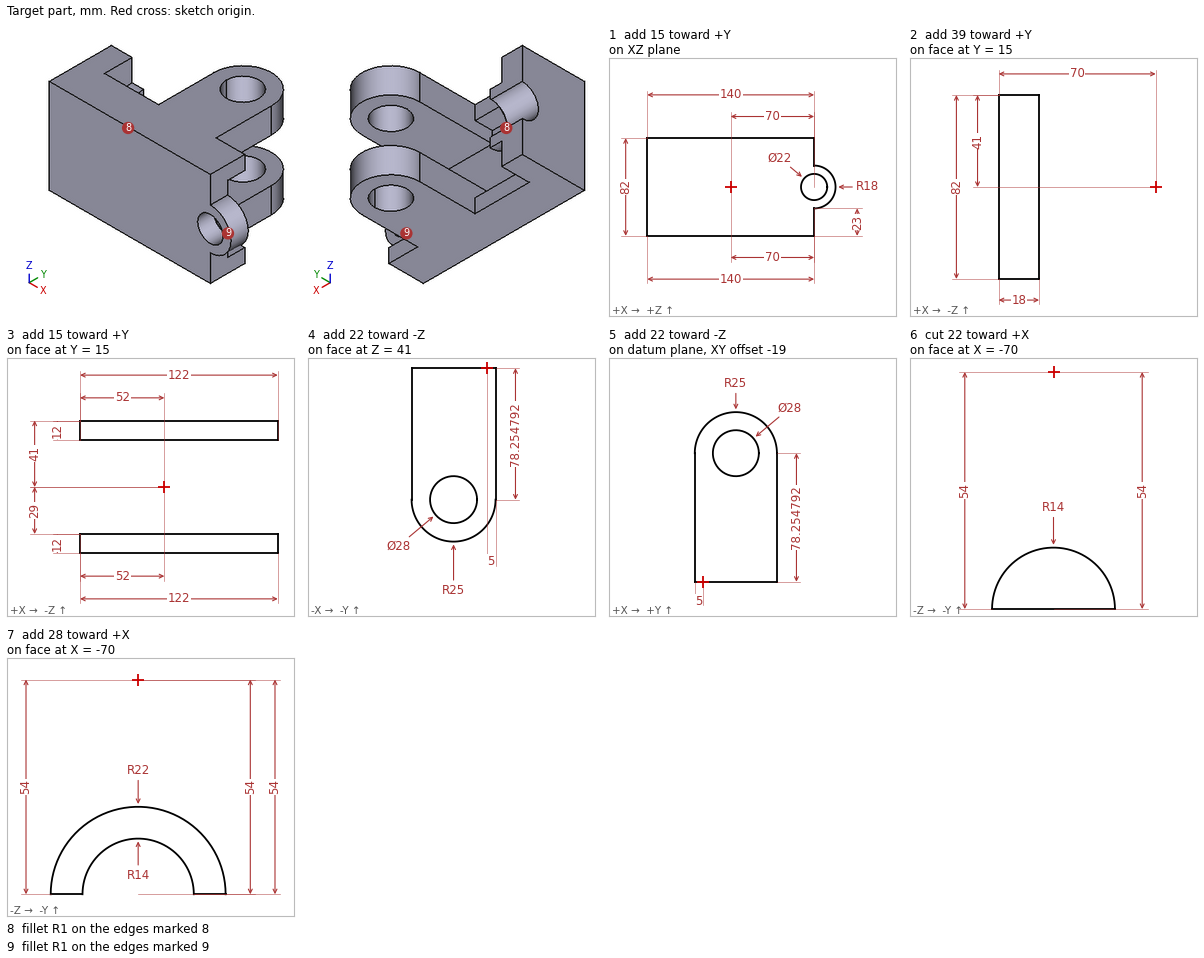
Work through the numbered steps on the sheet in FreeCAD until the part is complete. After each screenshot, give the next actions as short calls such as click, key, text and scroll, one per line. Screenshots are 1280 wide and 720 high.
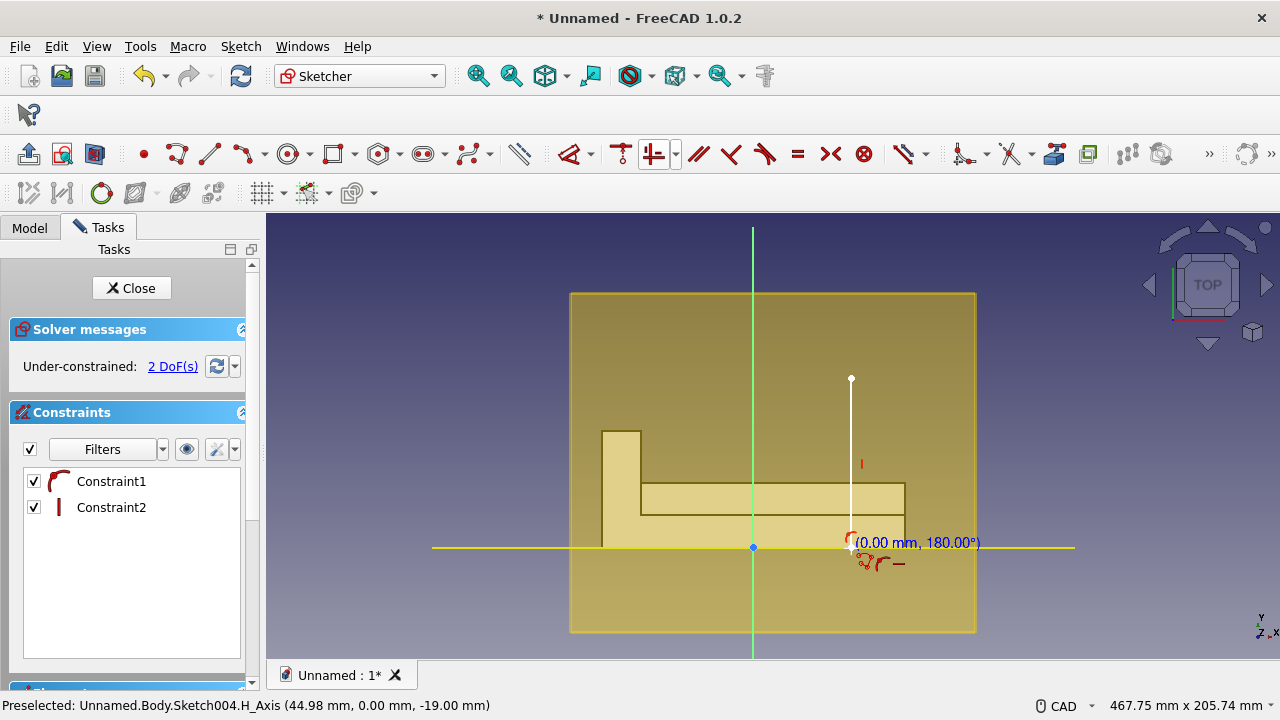
scroll(743, 548, up, 2)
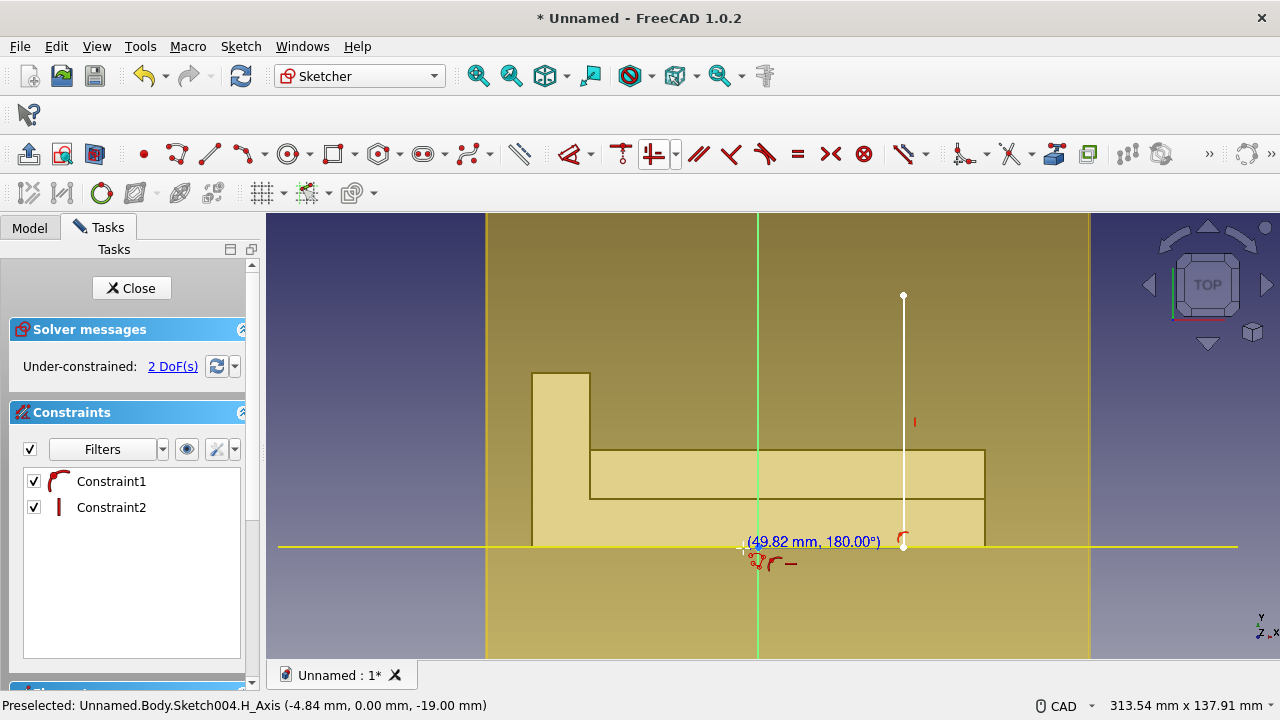
click(742, 538)
click(742, 294)
right_click(742, 294)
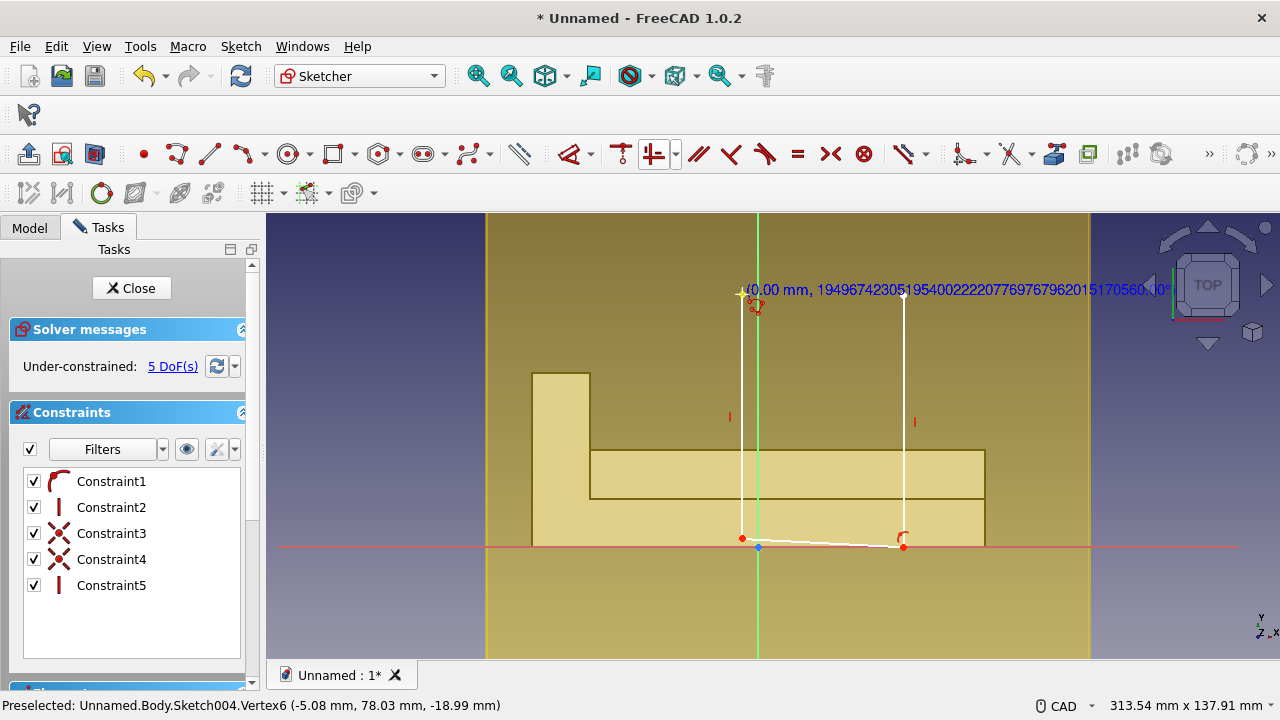
click(242, 154)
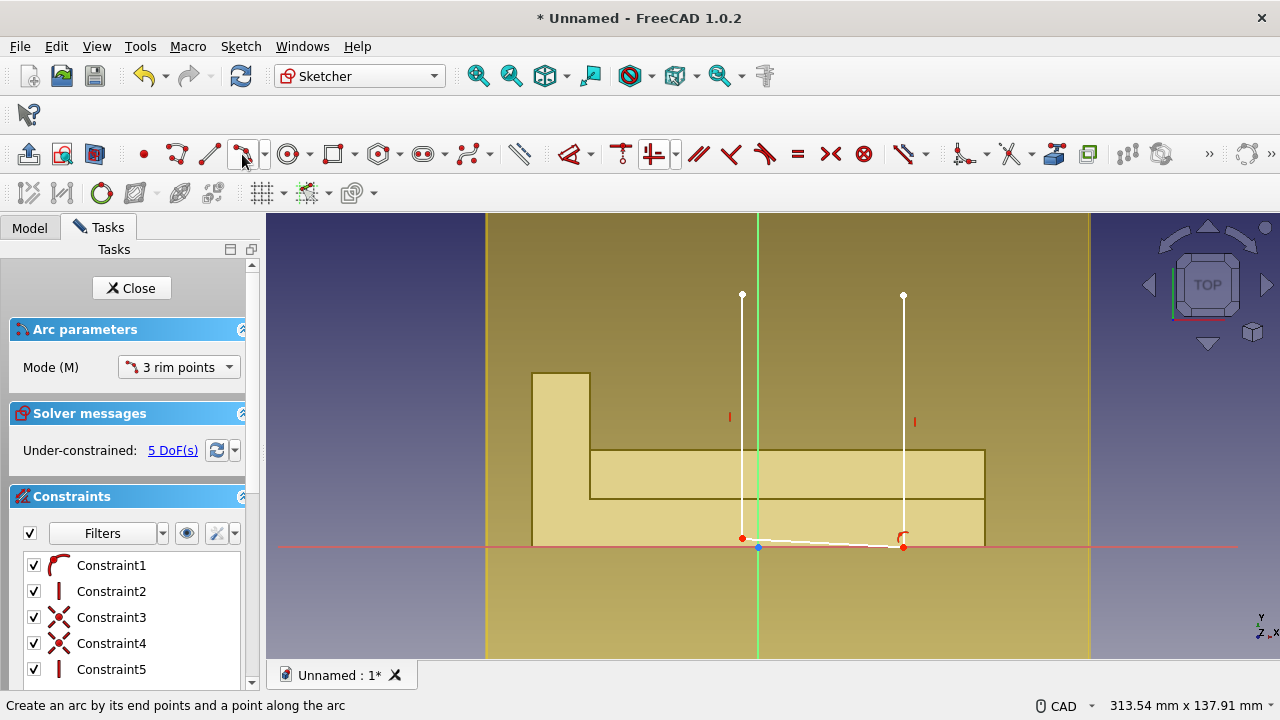
click(742, 295)
click(904, 296)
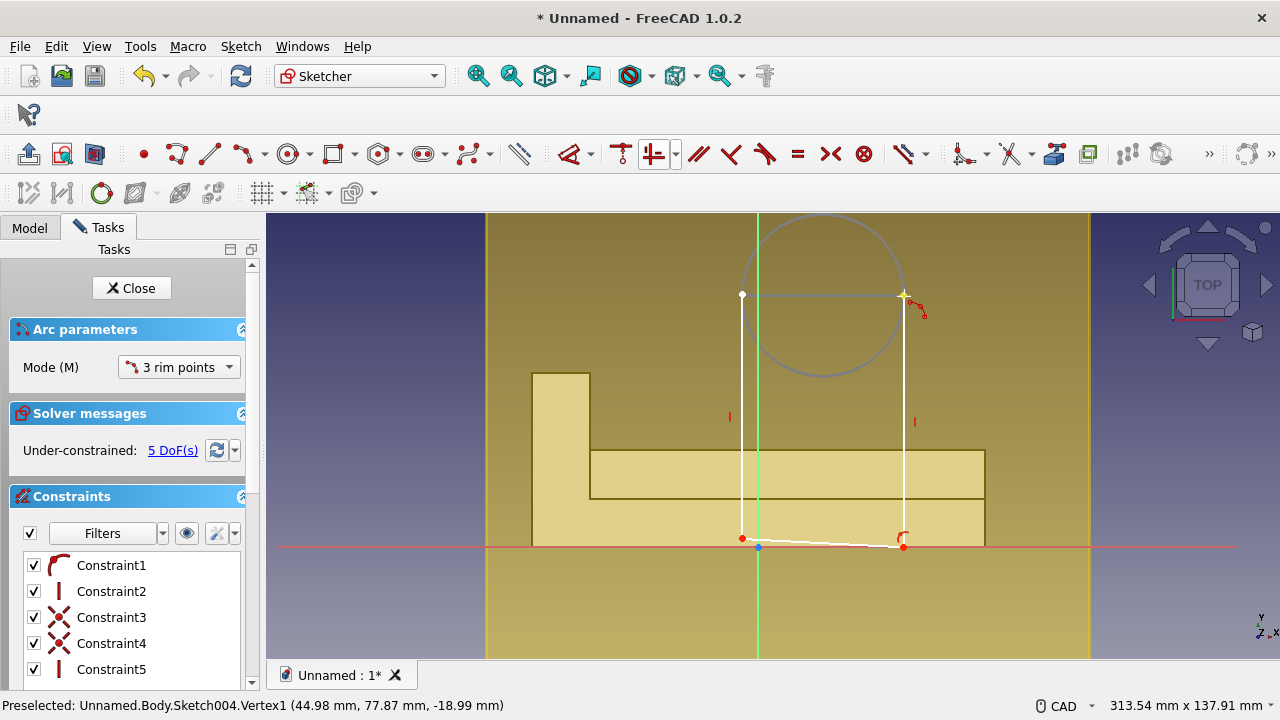
scroll(294, 631, down, 1)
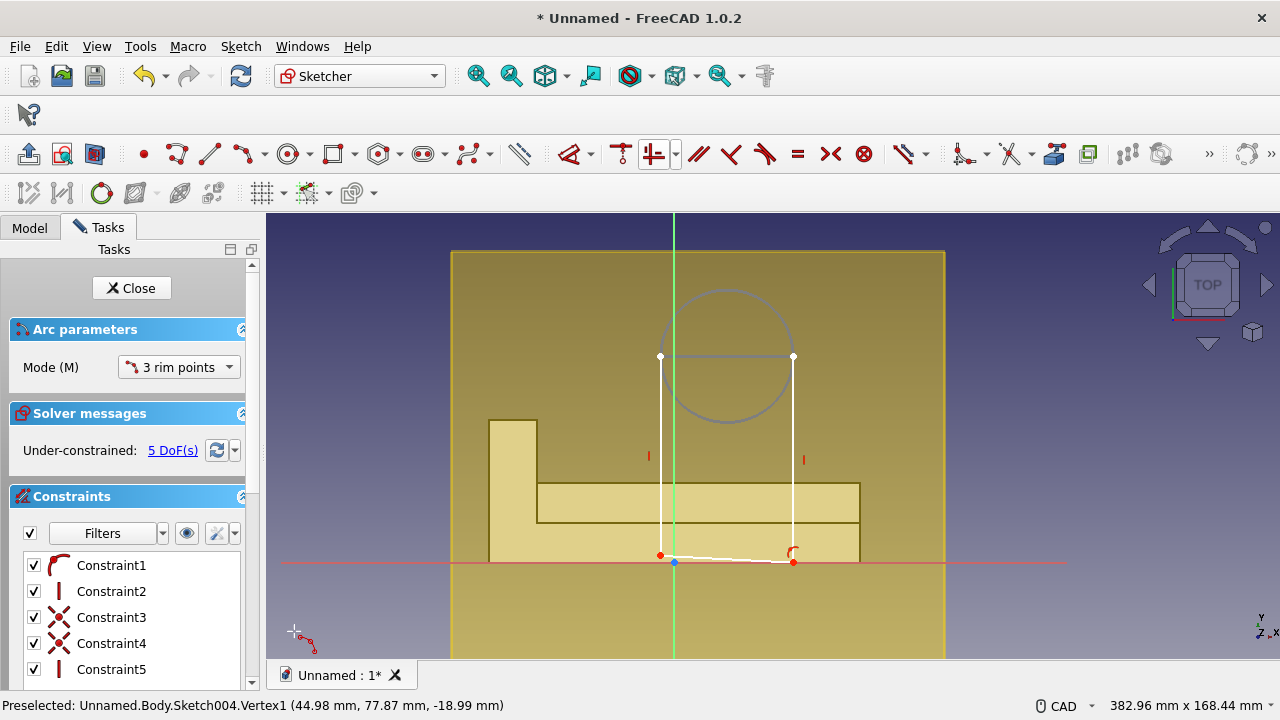
click(727, 289)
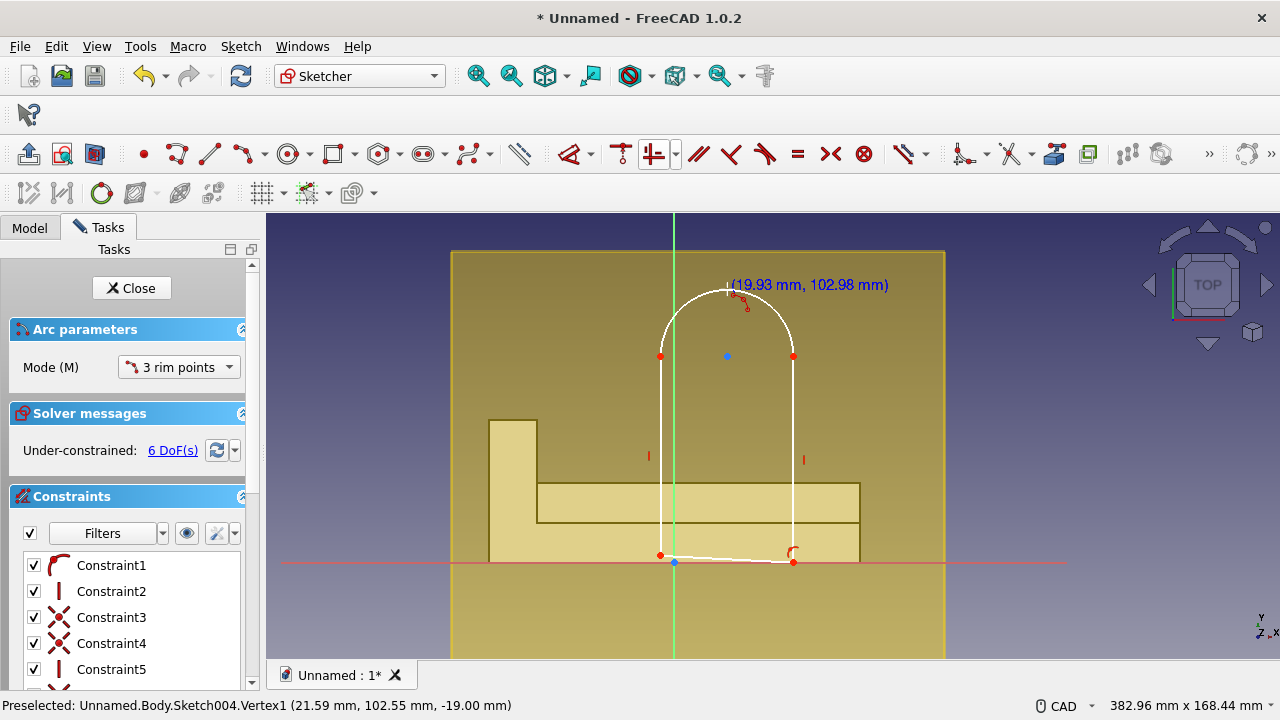
click(288, 154)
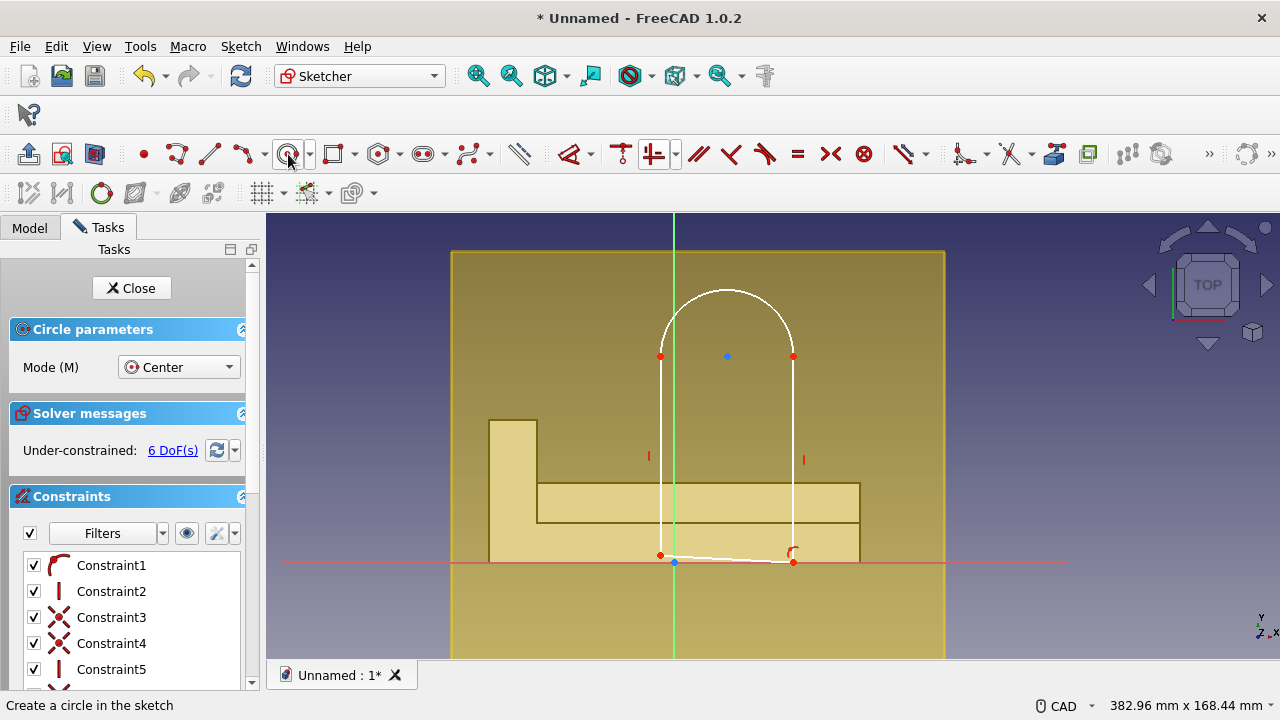
click(727, 355)
click(753, 329)
key(Escape)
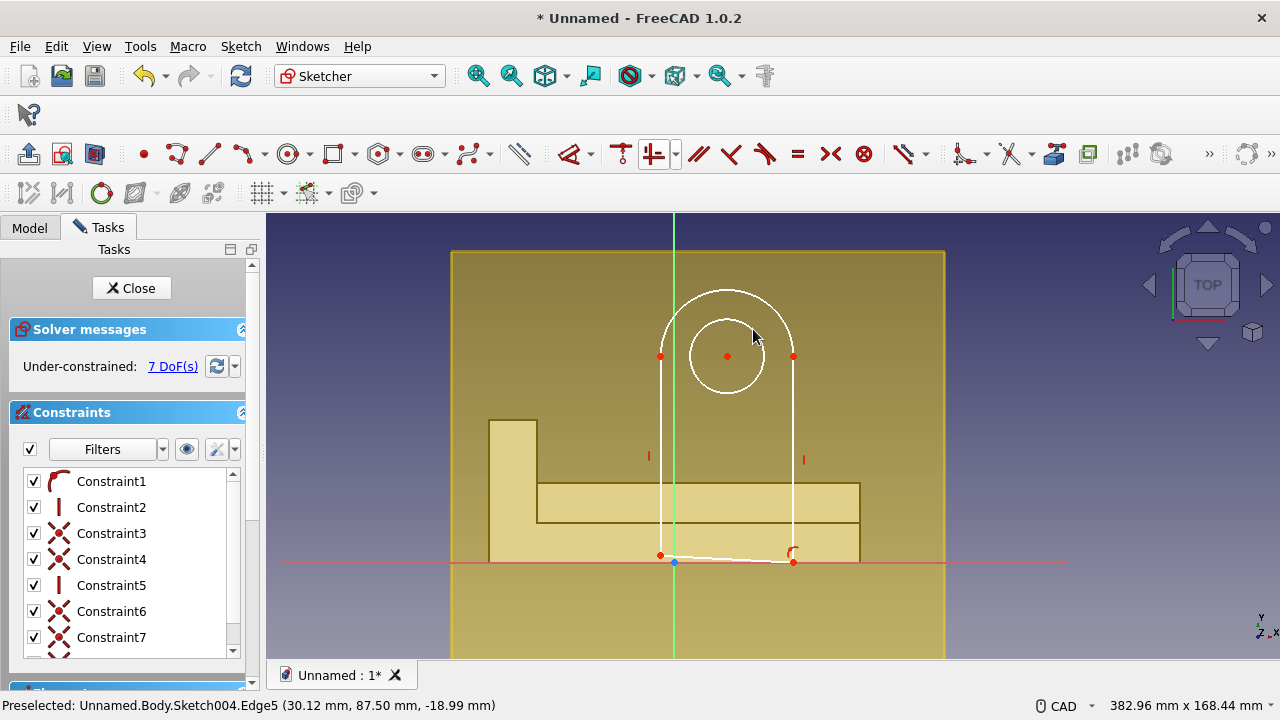
click(793, 418)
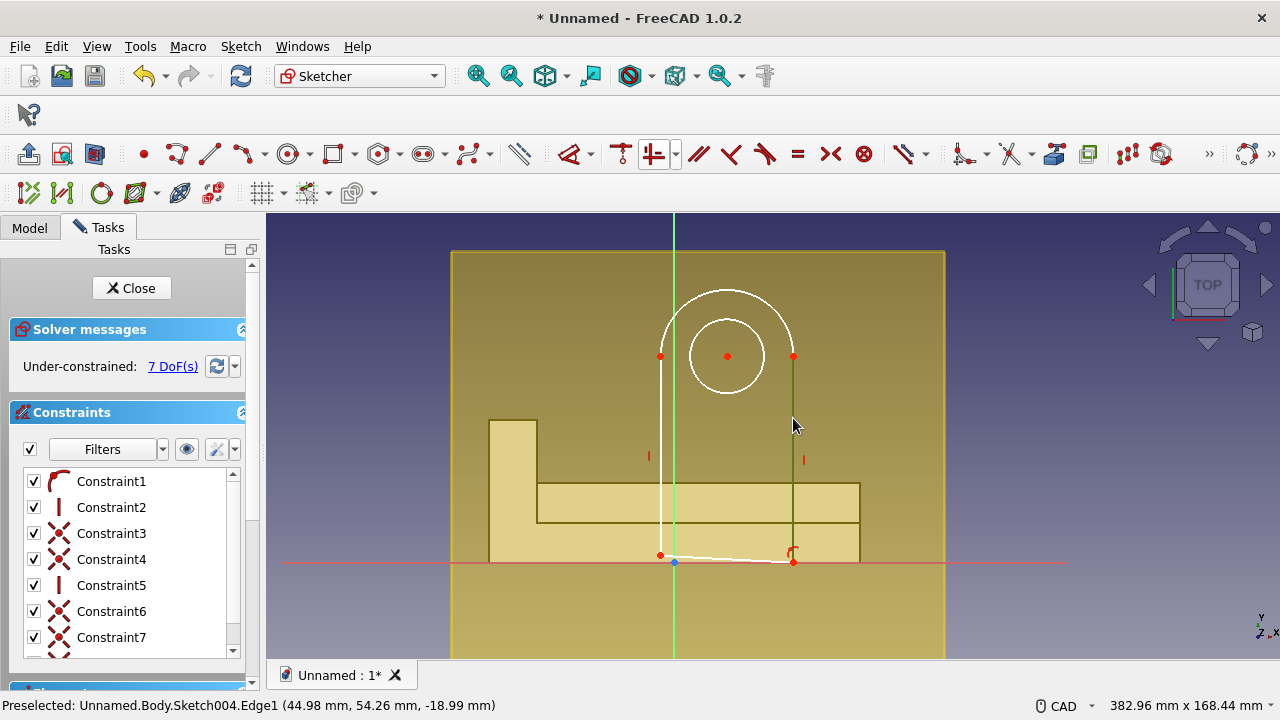
click(766, 303)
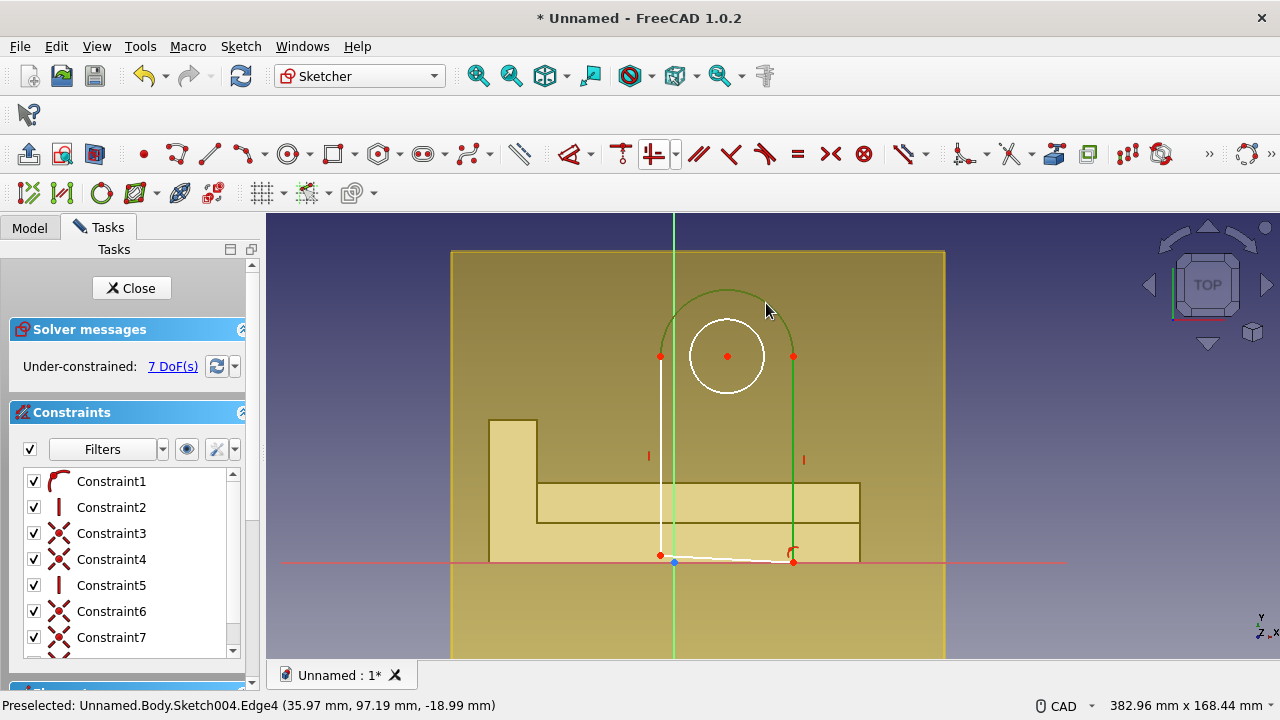
click(765, 154)